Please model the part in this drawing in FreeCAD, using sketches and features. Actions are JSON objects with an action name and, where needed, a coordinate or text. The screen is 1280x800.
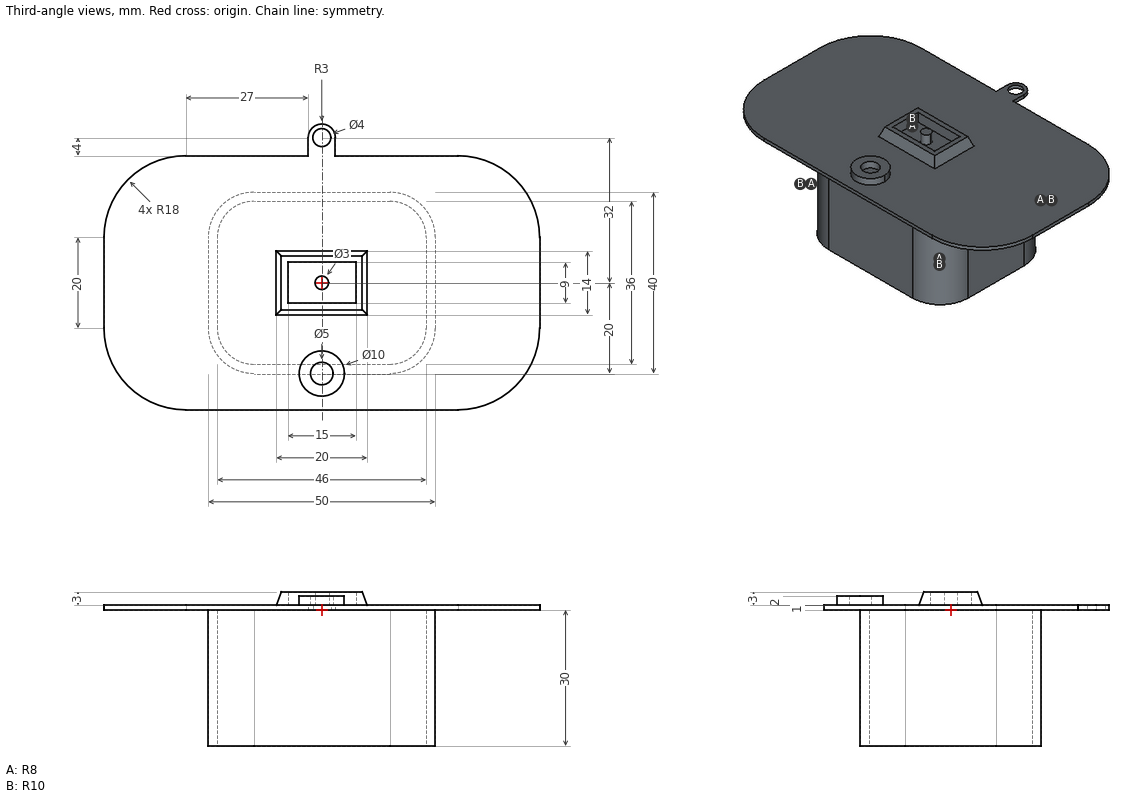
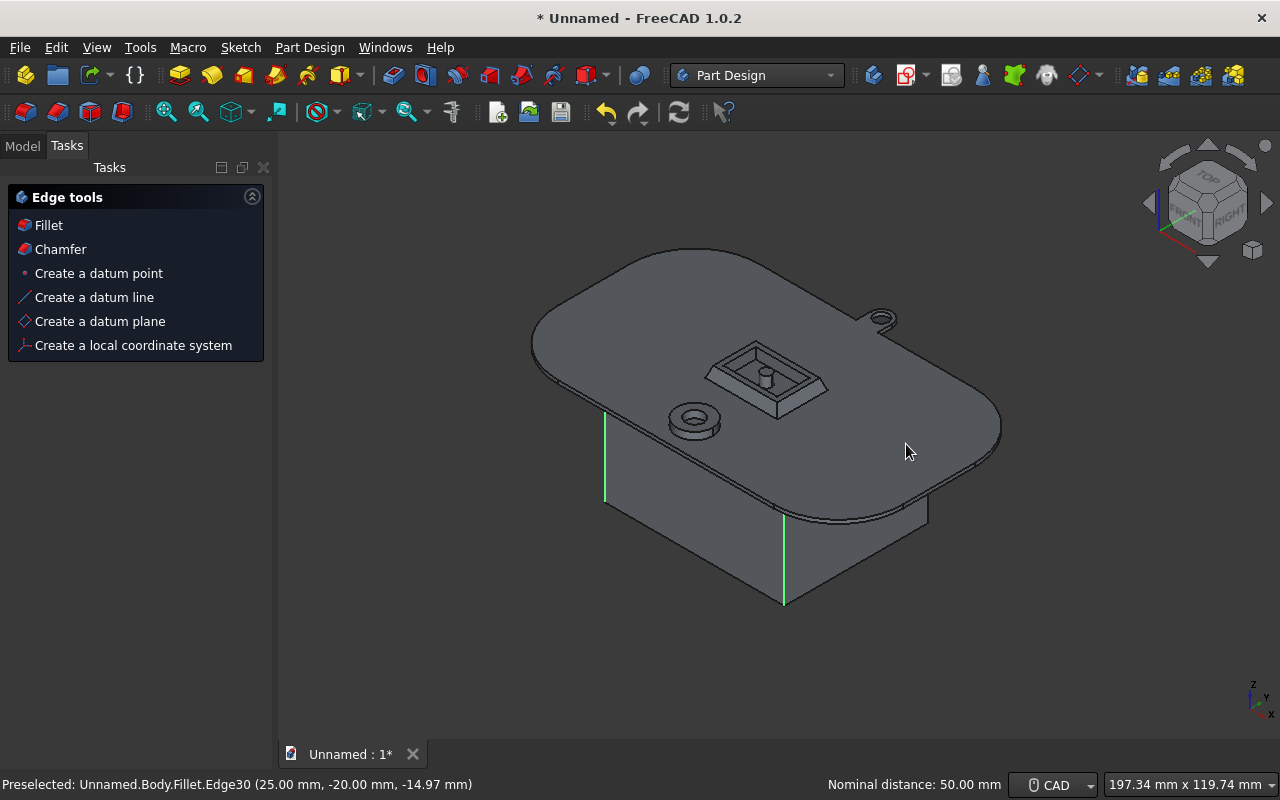
{"action": "key", "text": "2"}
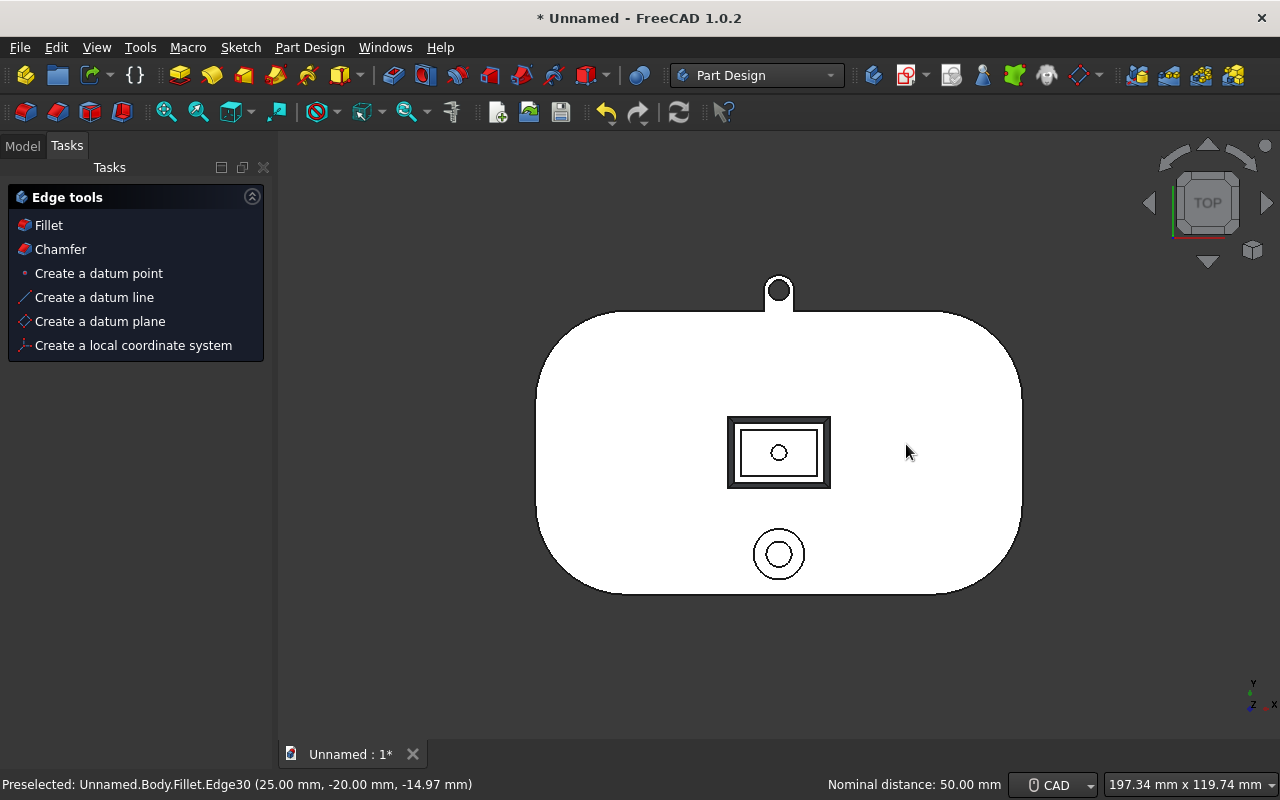
{"action": "key", "text": "1"}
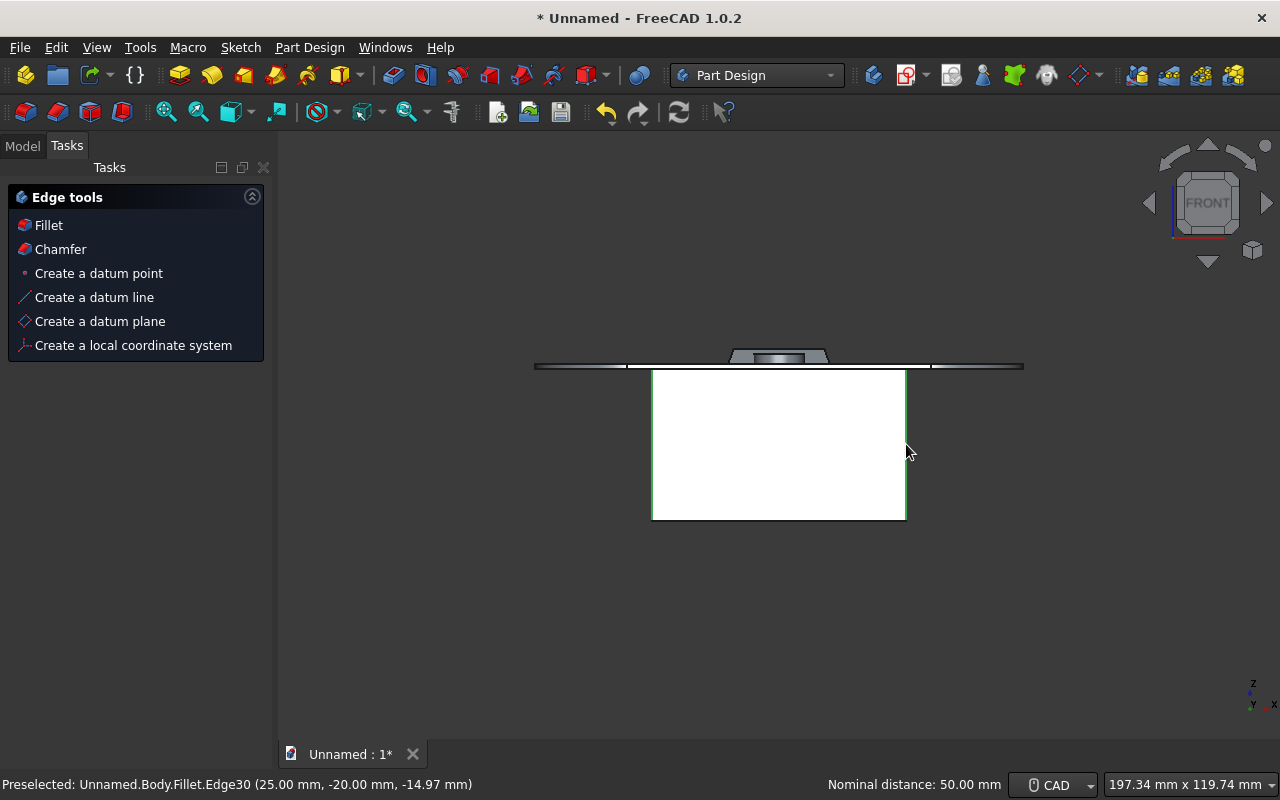
{"action": "key", "text": "3"}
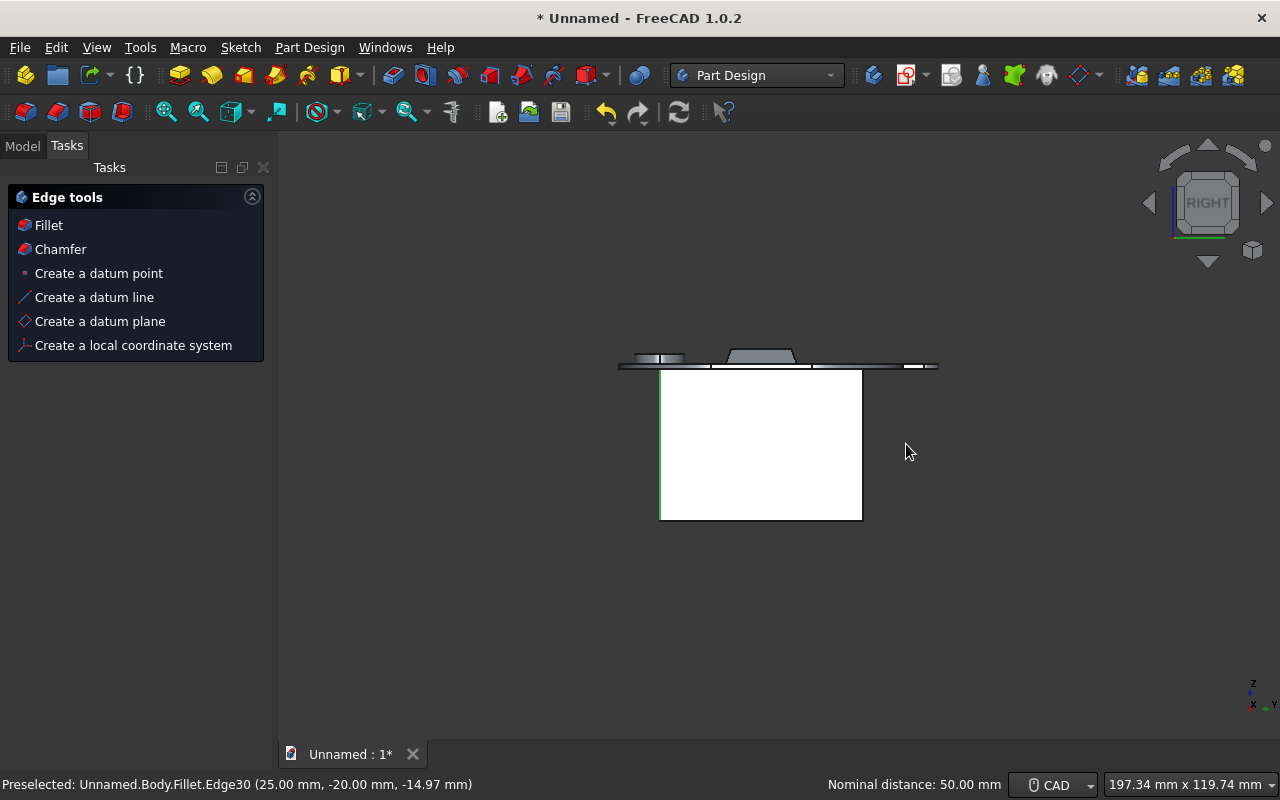
{"action": "left_click", "coordinate": [168, 112]}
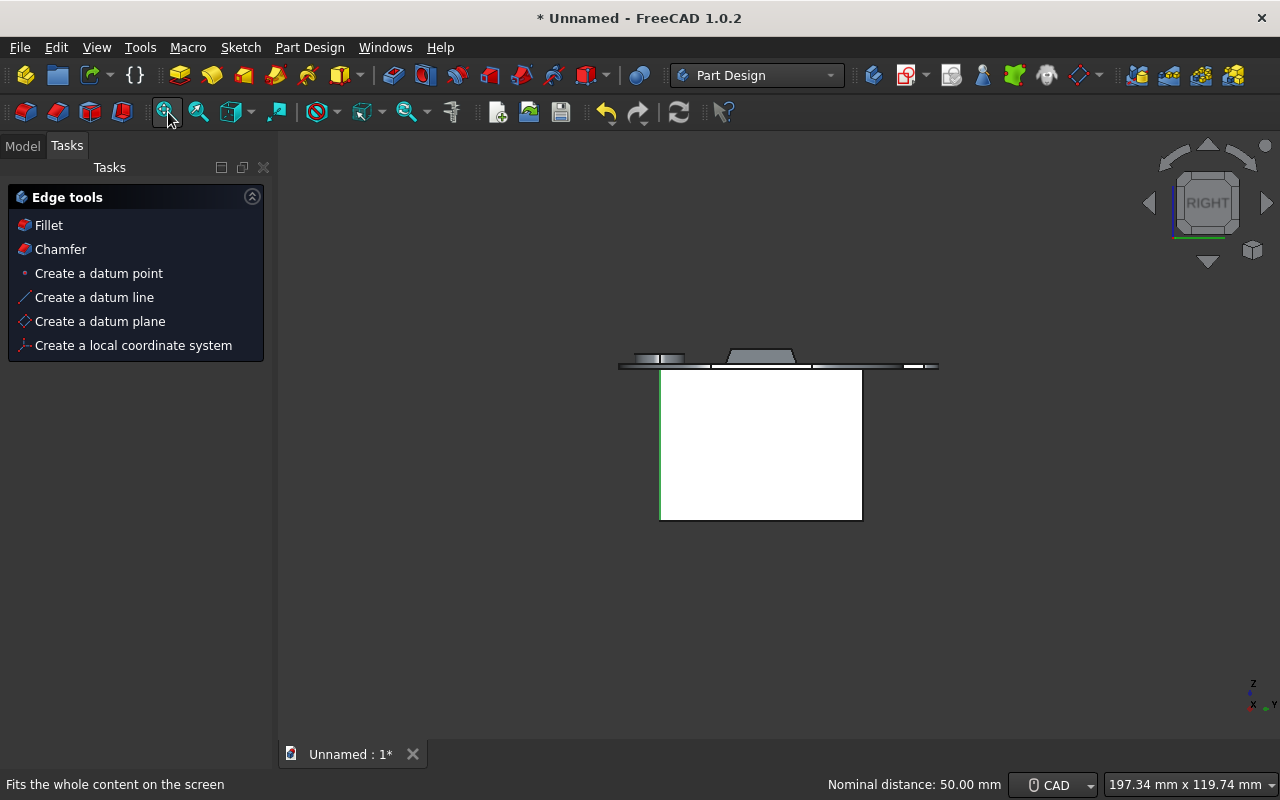
{"action": "left_click", "coordinate": [863, 444], "text": "ctrl"}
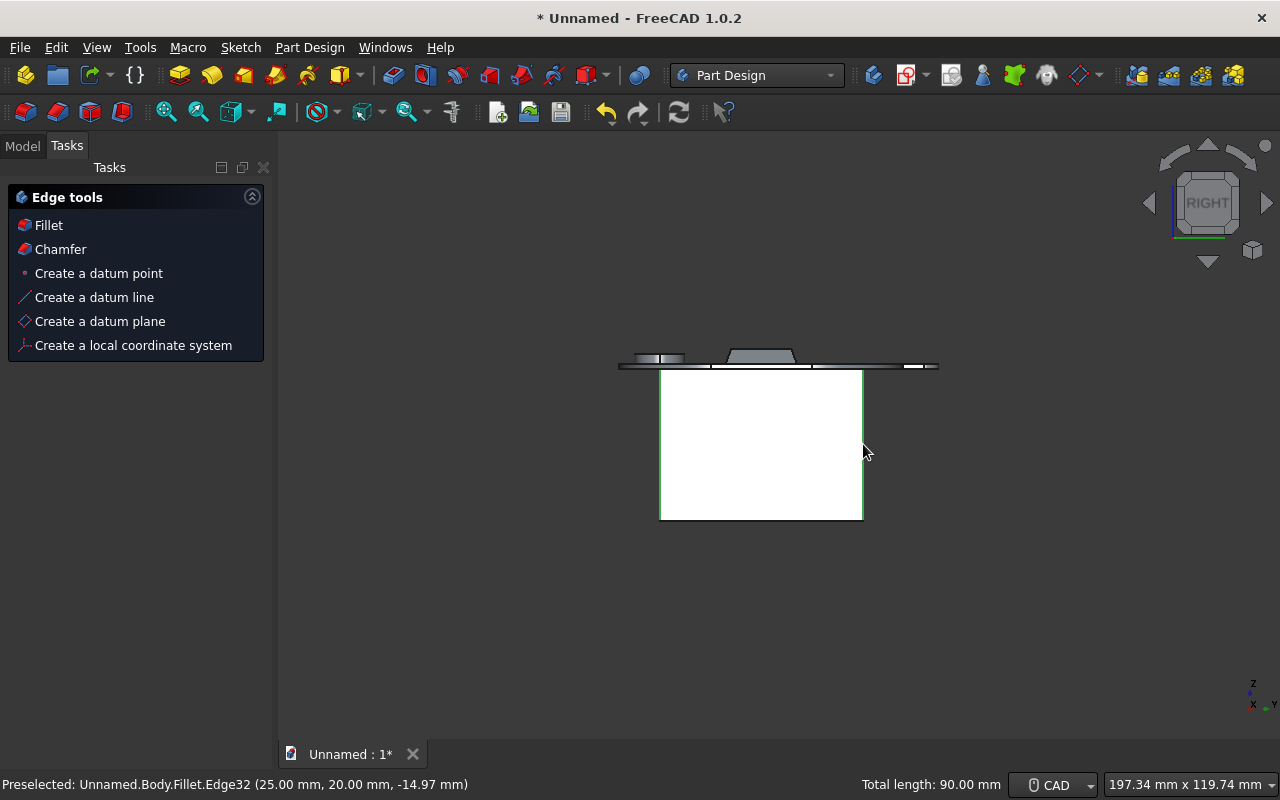
{"action": "key", "text": "5"}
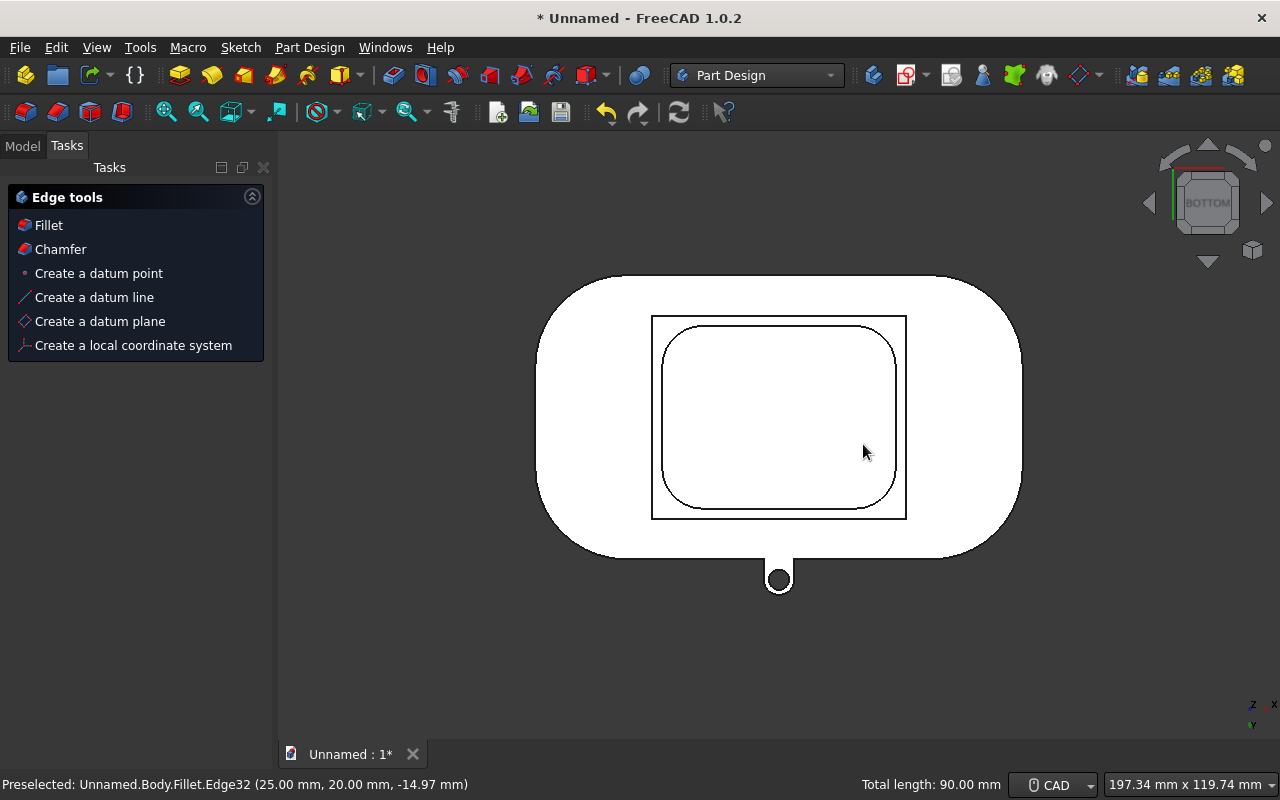
{"action": "key", "text": "4"}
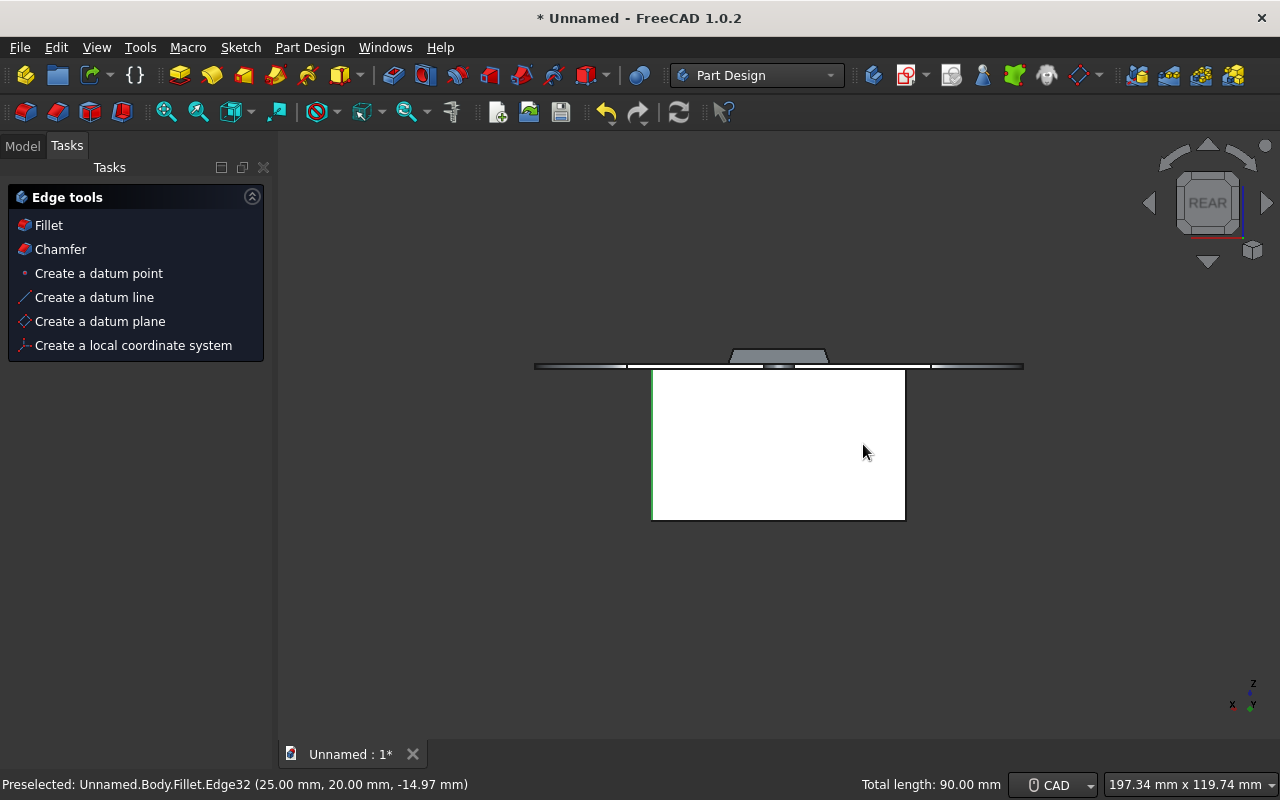
{"action": "left_click", "coordinate": [906, 444], "text": "ctrl"}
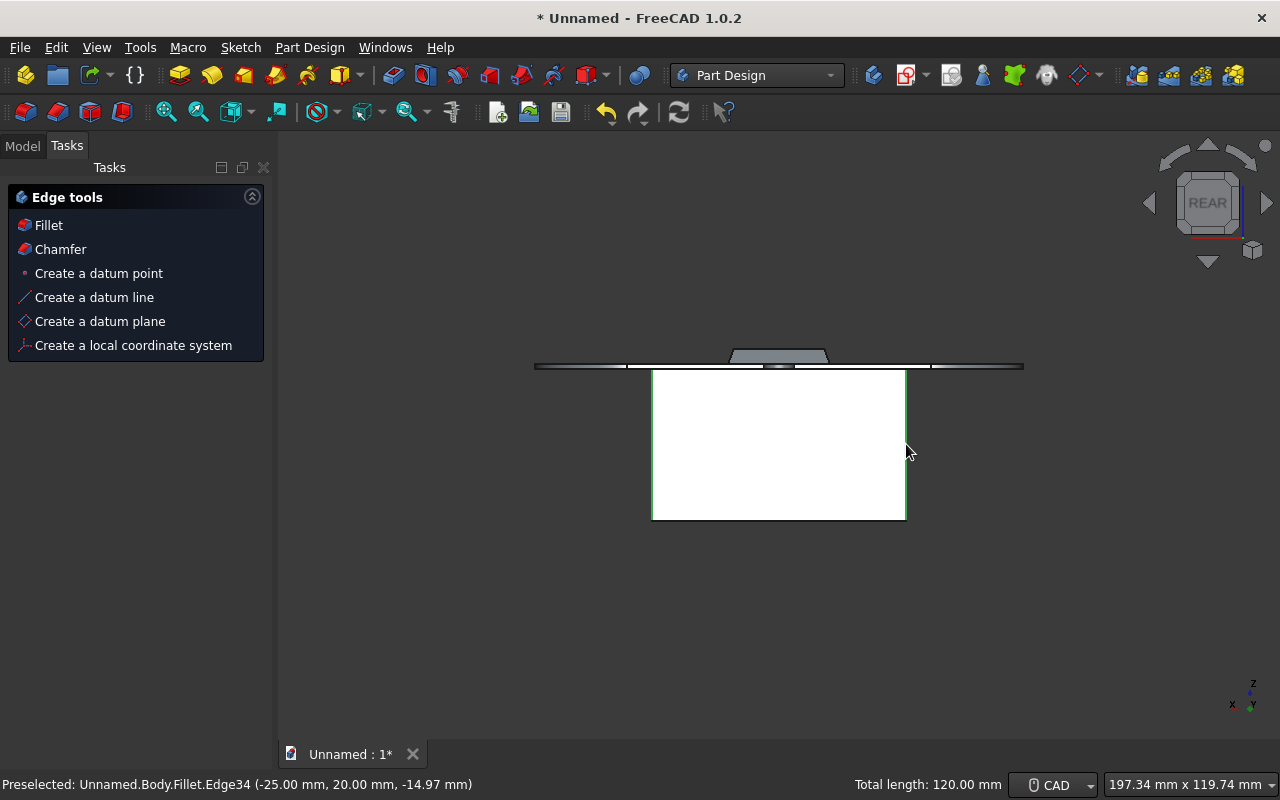
{"action": "left_click", "coordinate": [26, 112]}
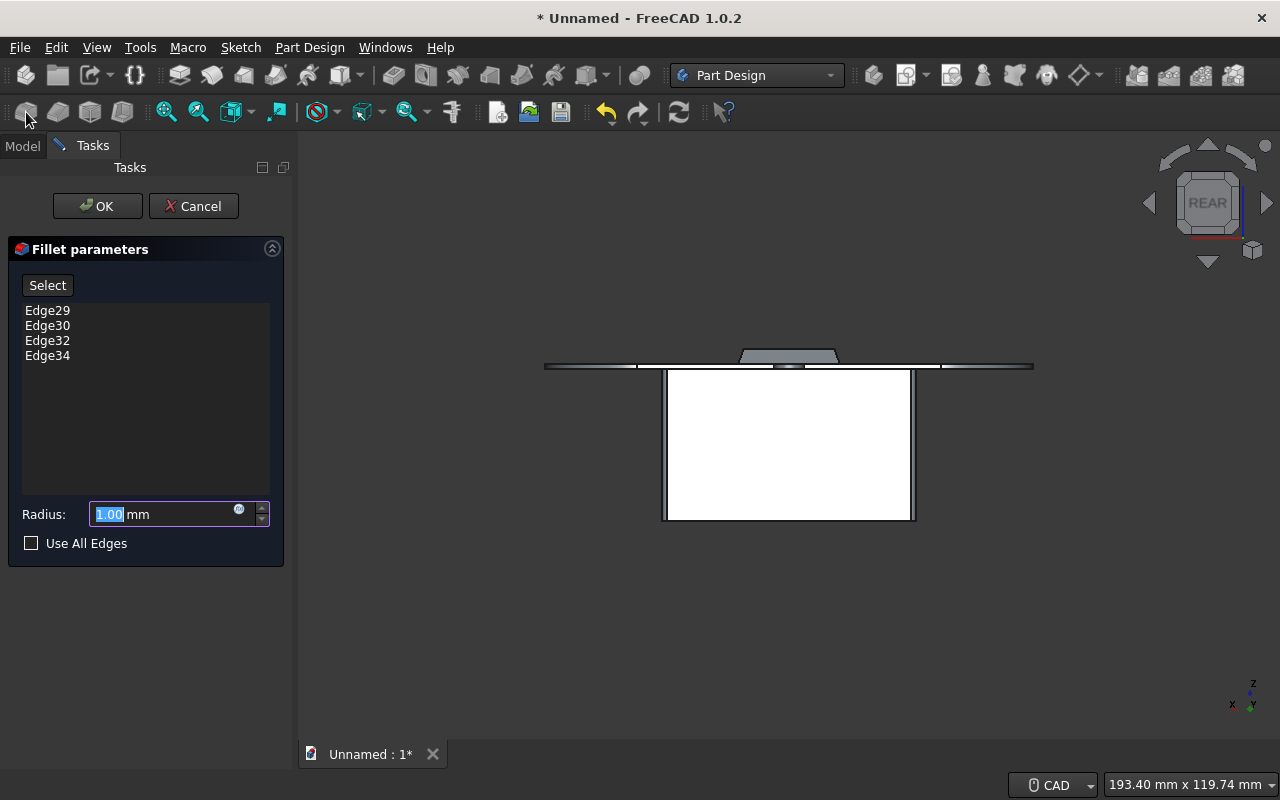
{"action": "type", "text": "10"}
{"action": "key", "text": "Tab"}